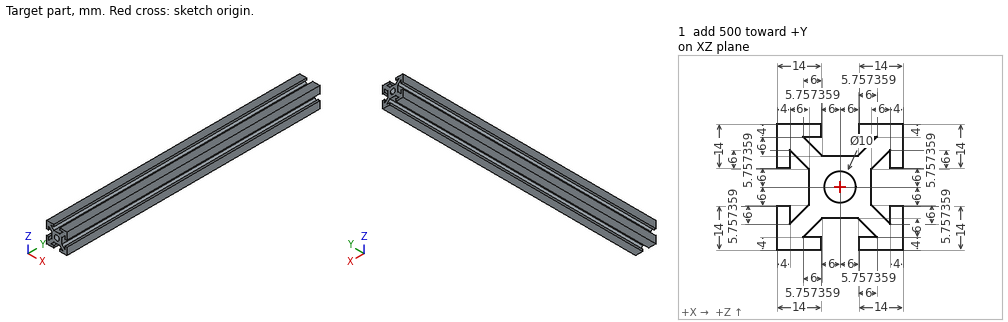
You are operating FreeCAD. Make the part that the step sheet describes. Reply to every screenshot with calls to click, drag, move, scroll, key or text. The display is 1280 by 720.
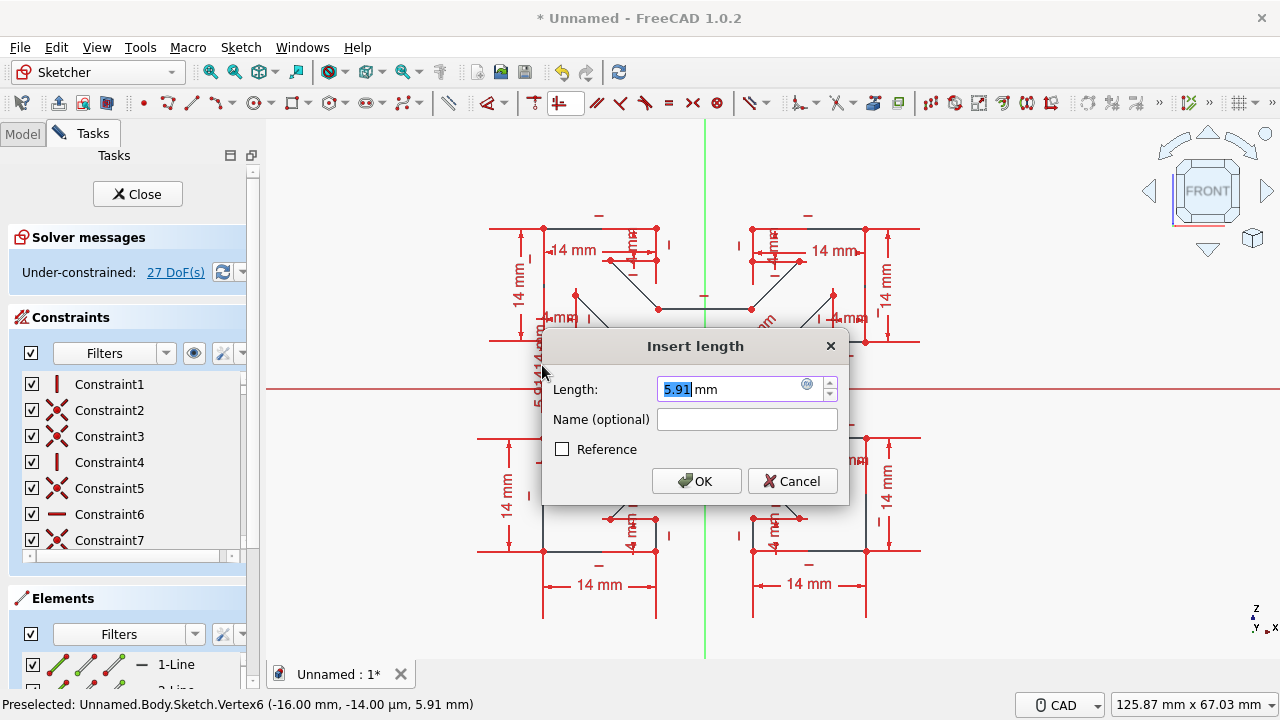
text(6)
key(Return)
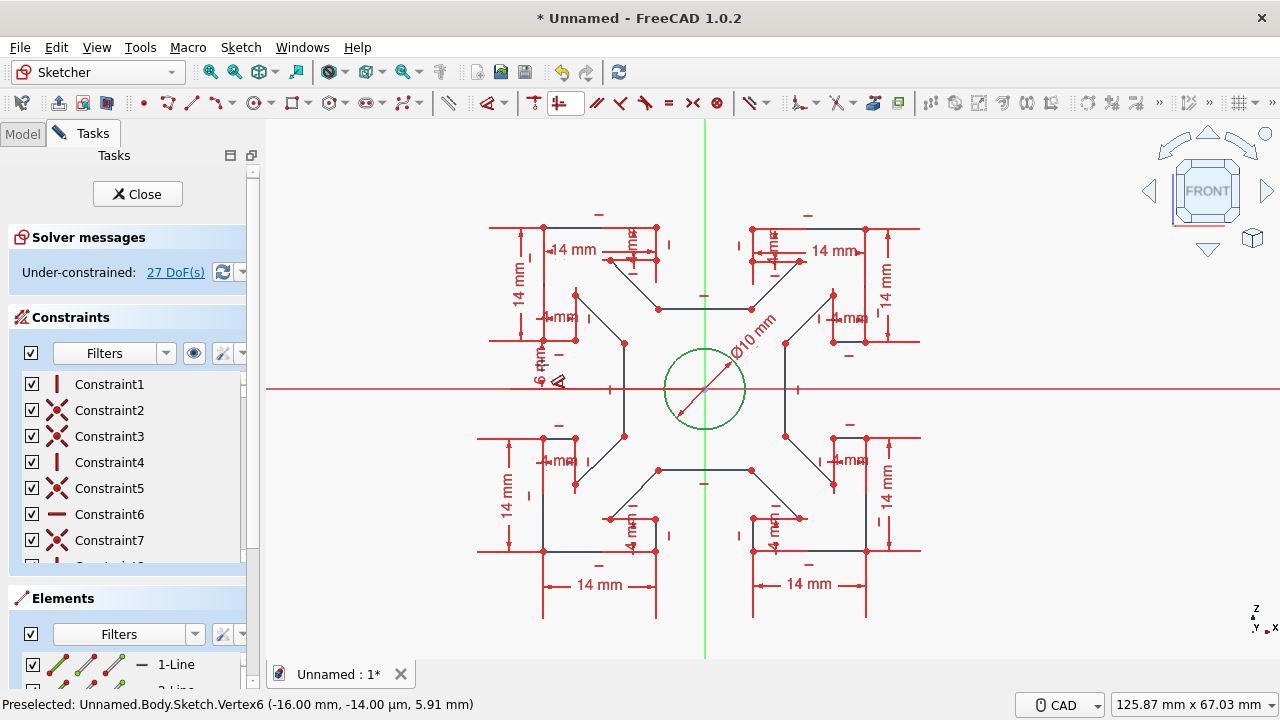
click(656, 228)
click(680, 194)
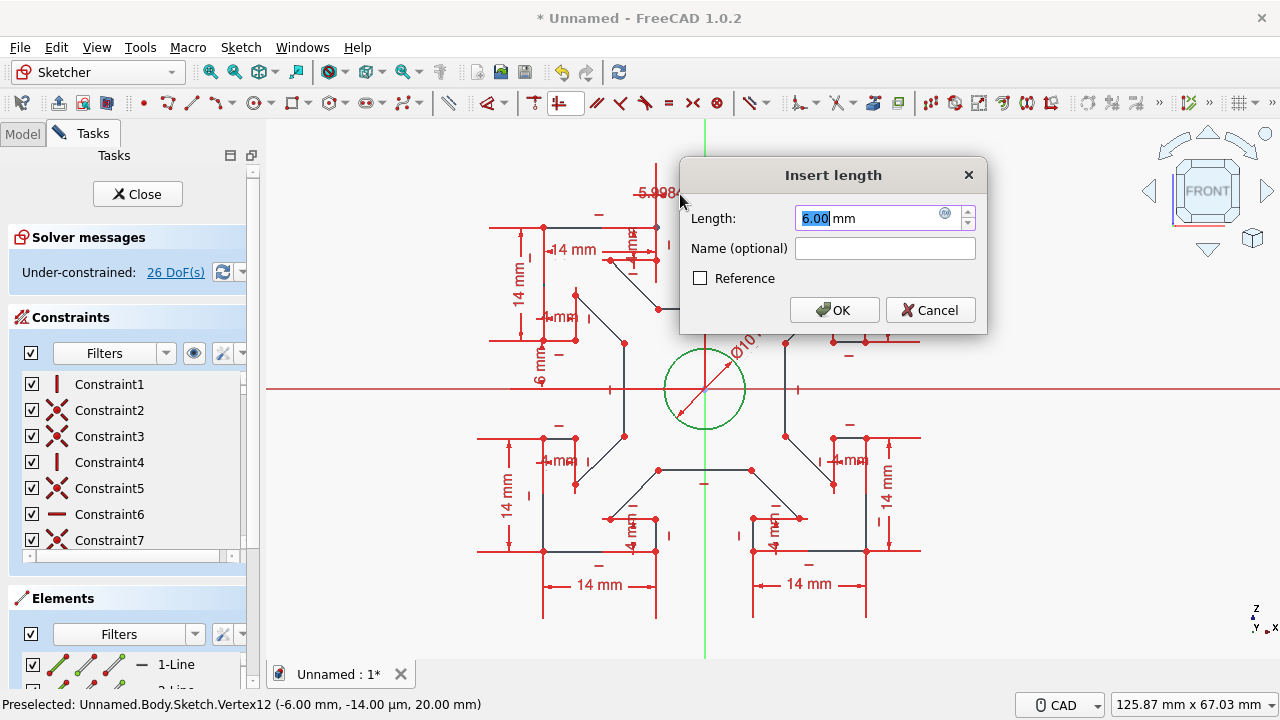
text(6)
key(Return)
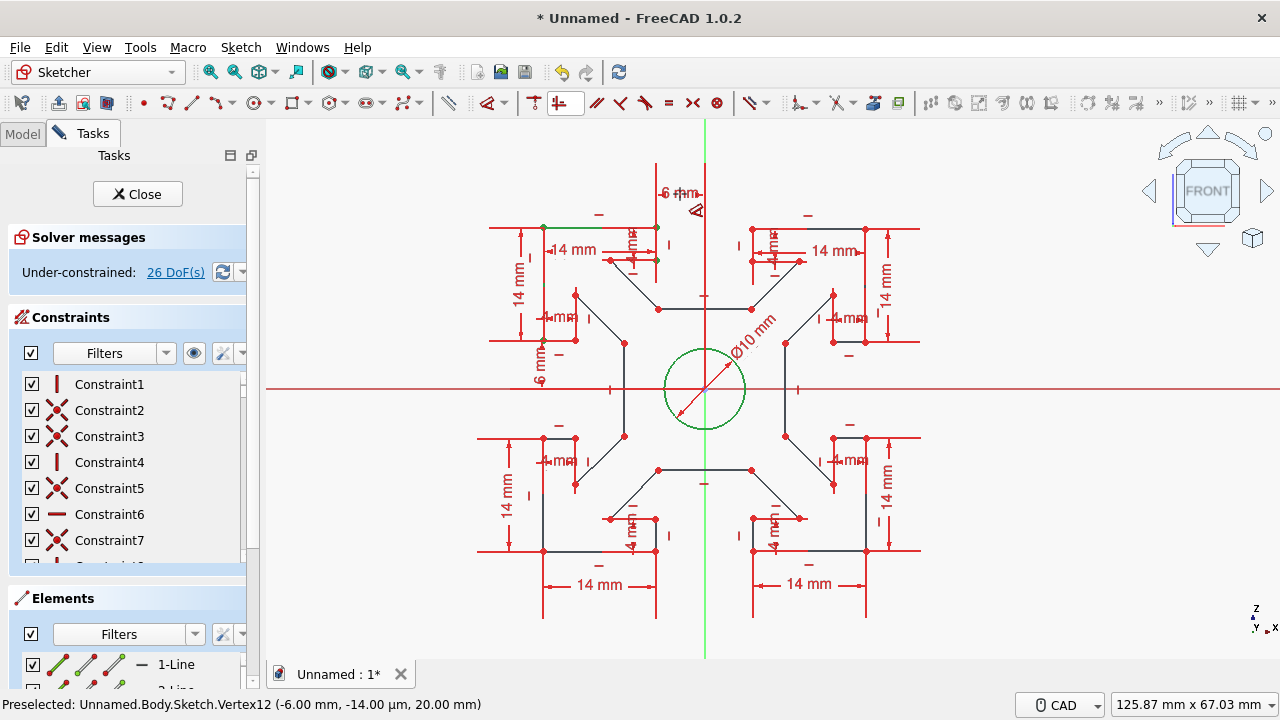
click(753, 262)
click(729, 447)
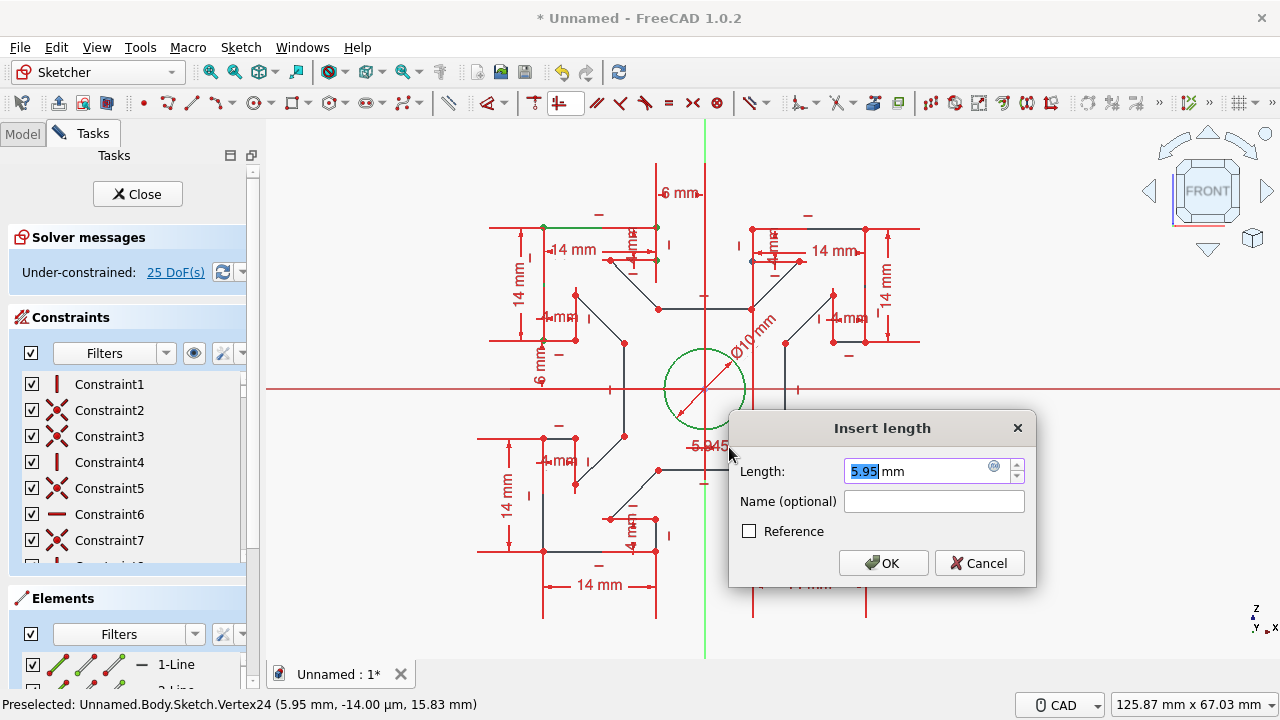
text(6)
key(Return)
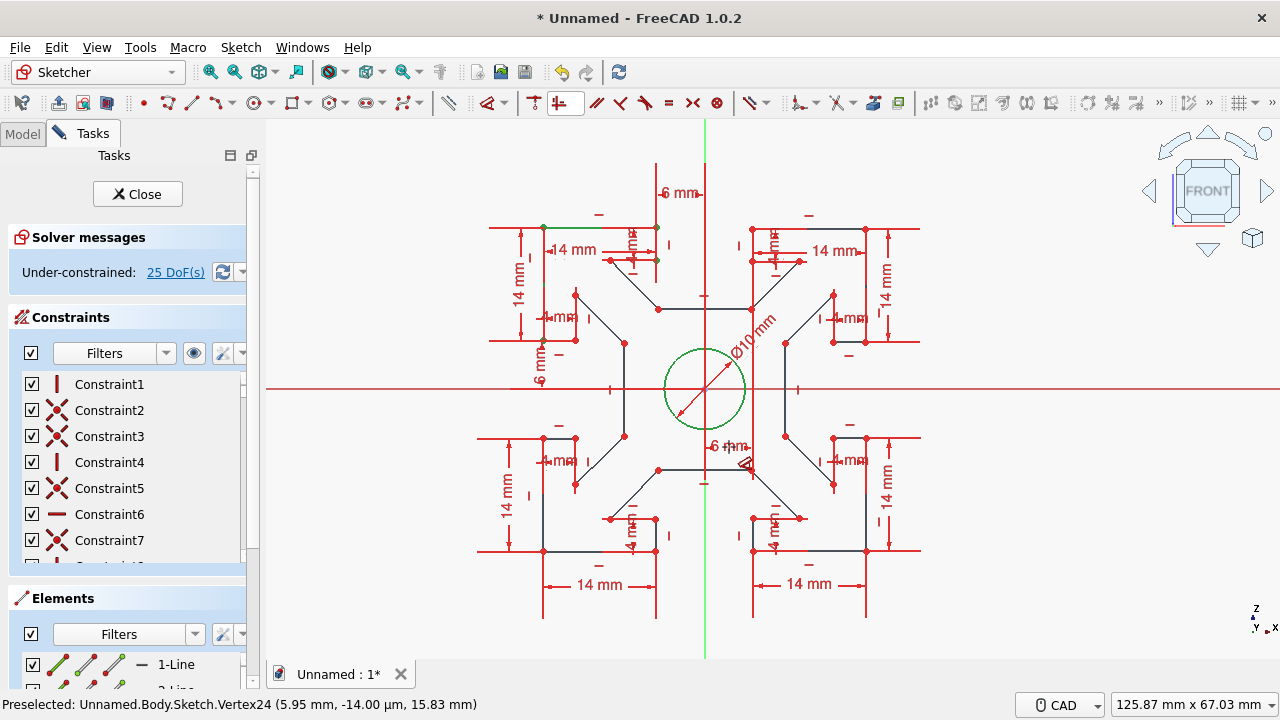
click(866, 342)
click(900, 366)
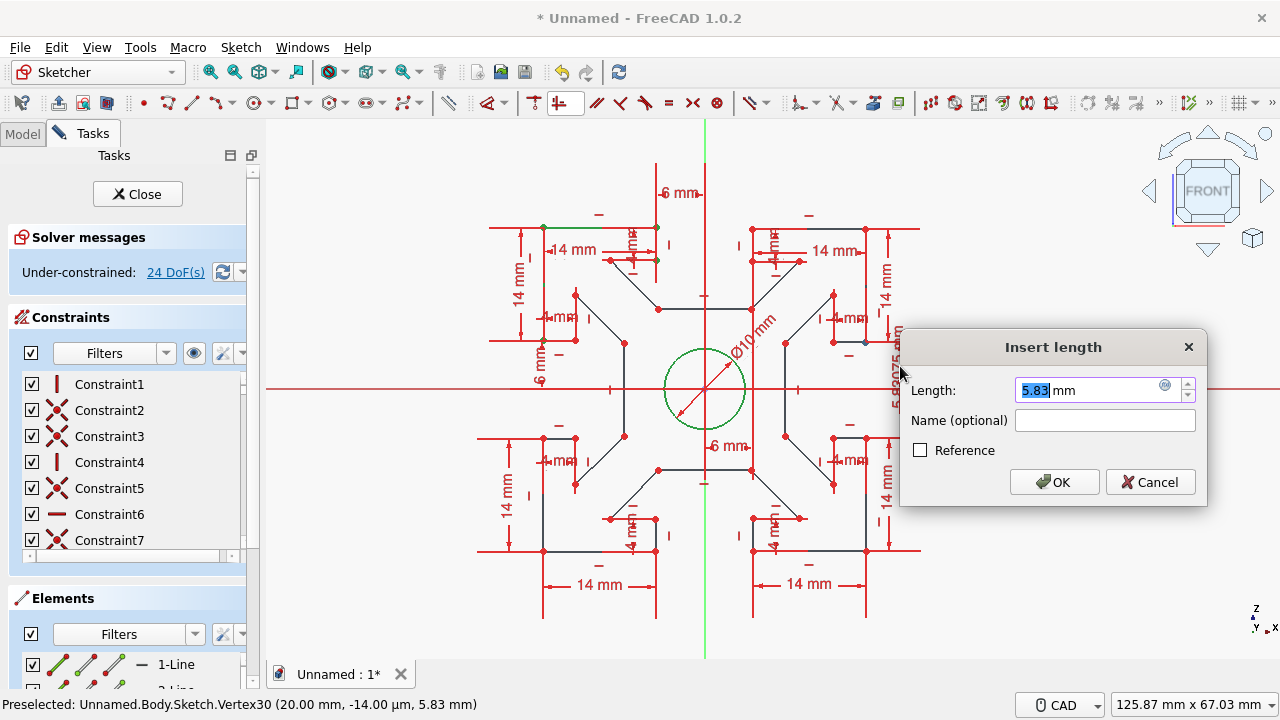
text(6)
key(Return)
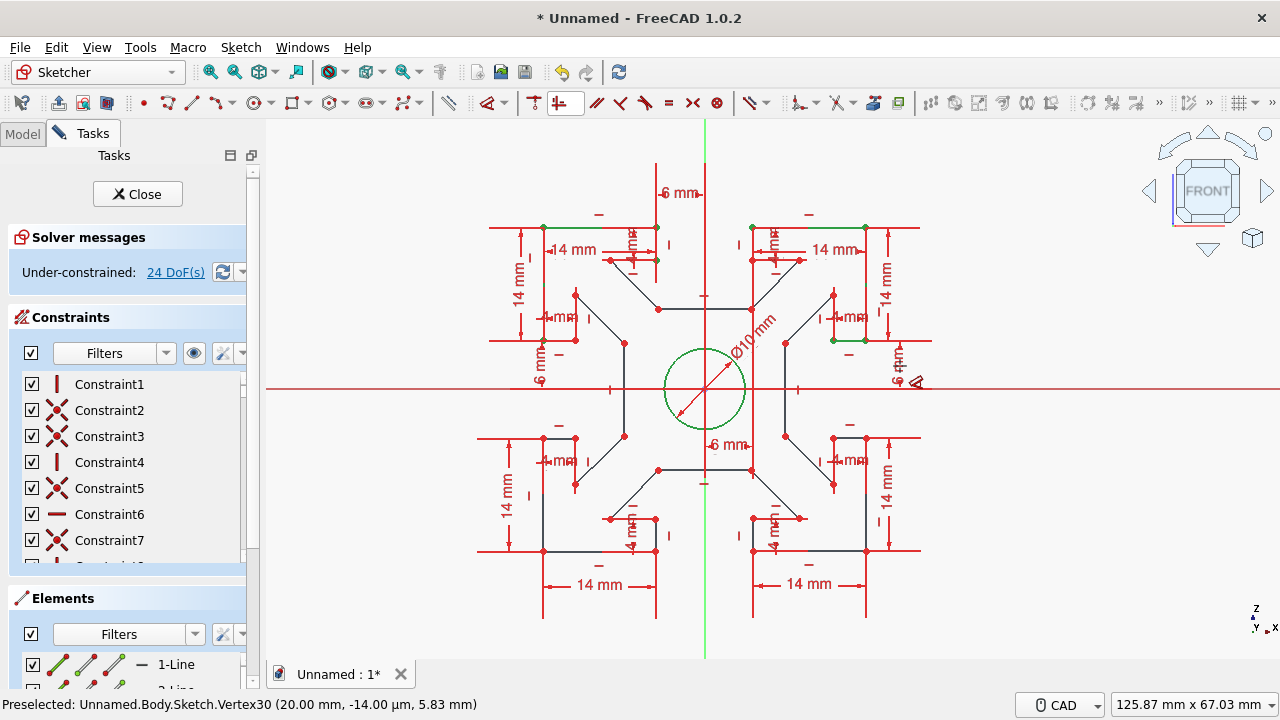
click(834, 438)
click(868, 414)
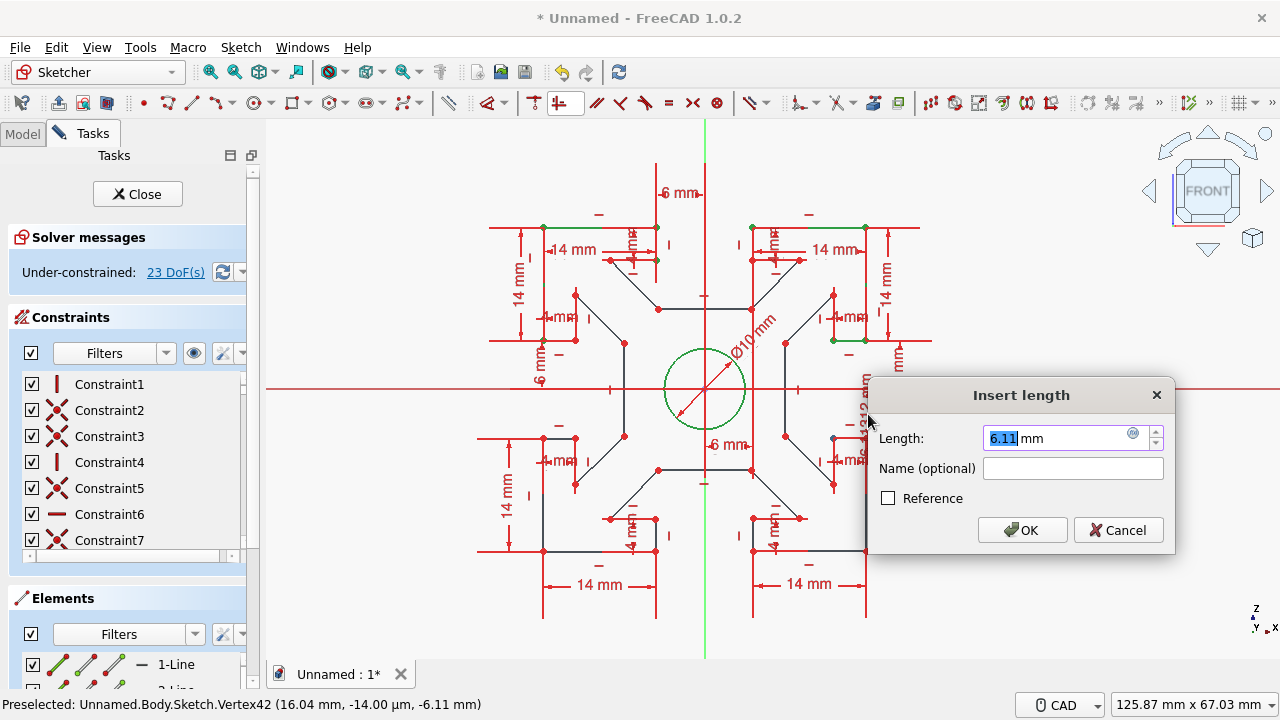
text(6)
key(Return)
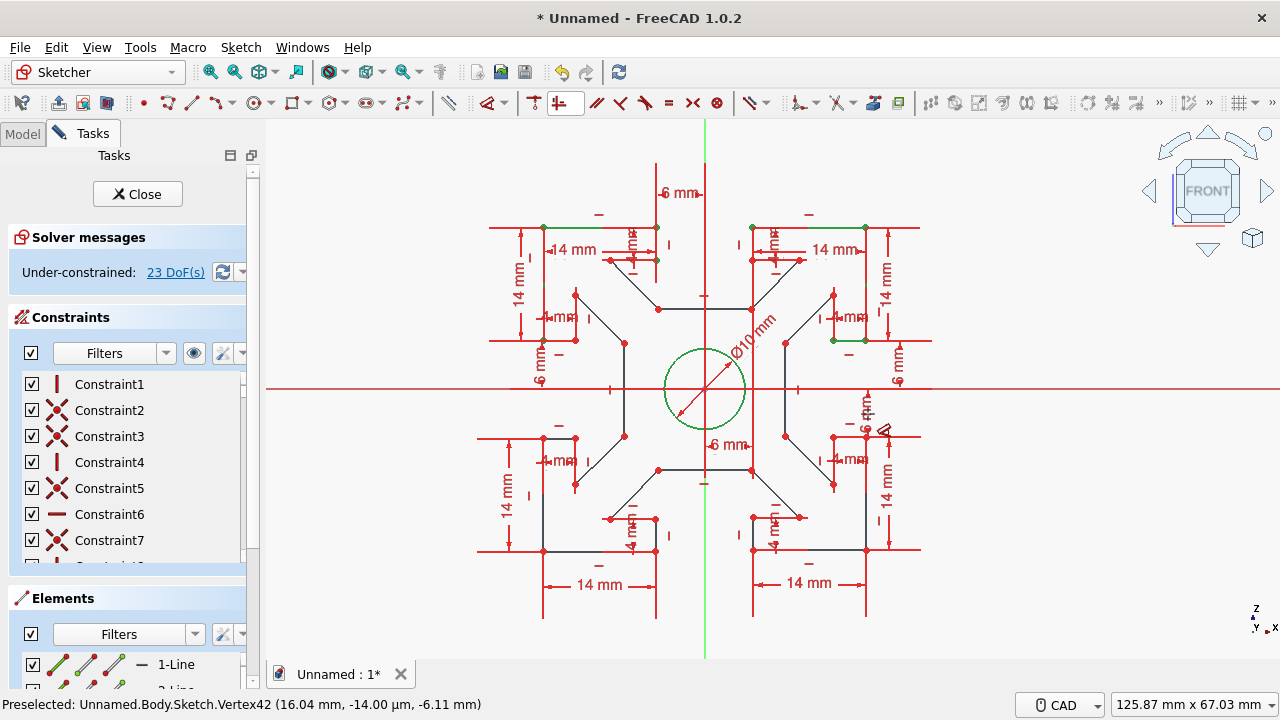
click(753, 550)
click(729, 584)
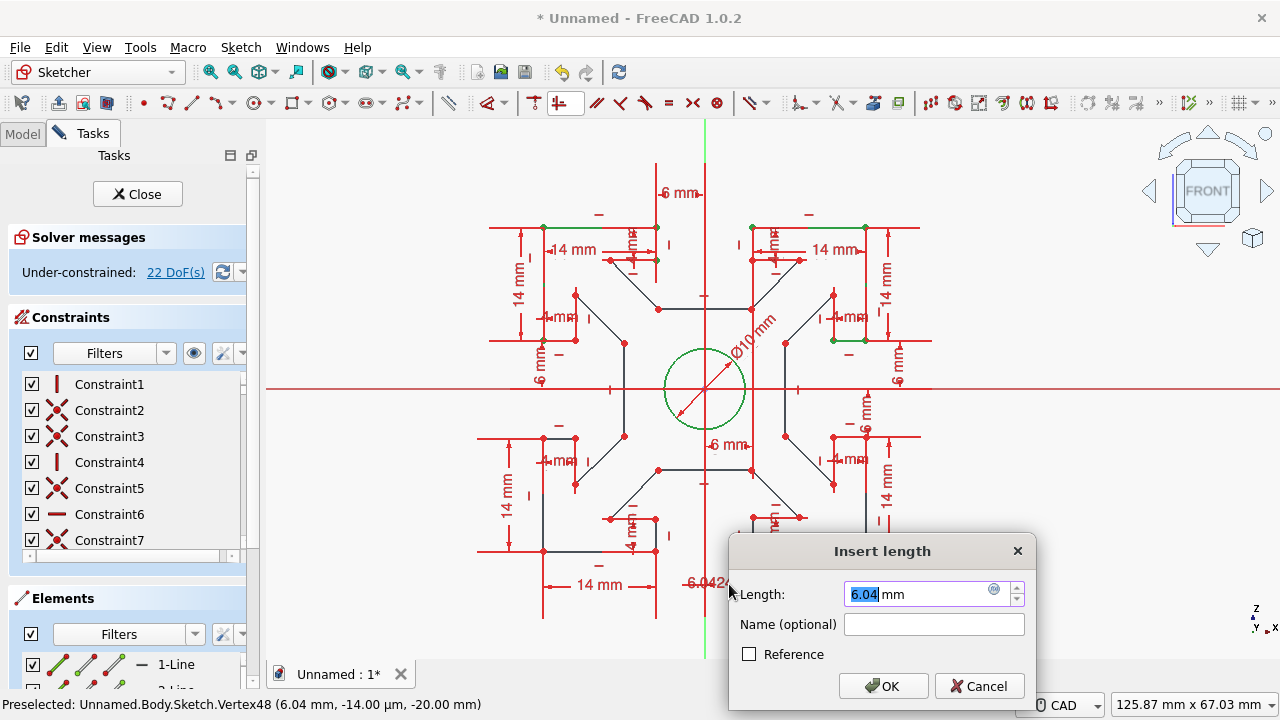
text(6)
key(Return)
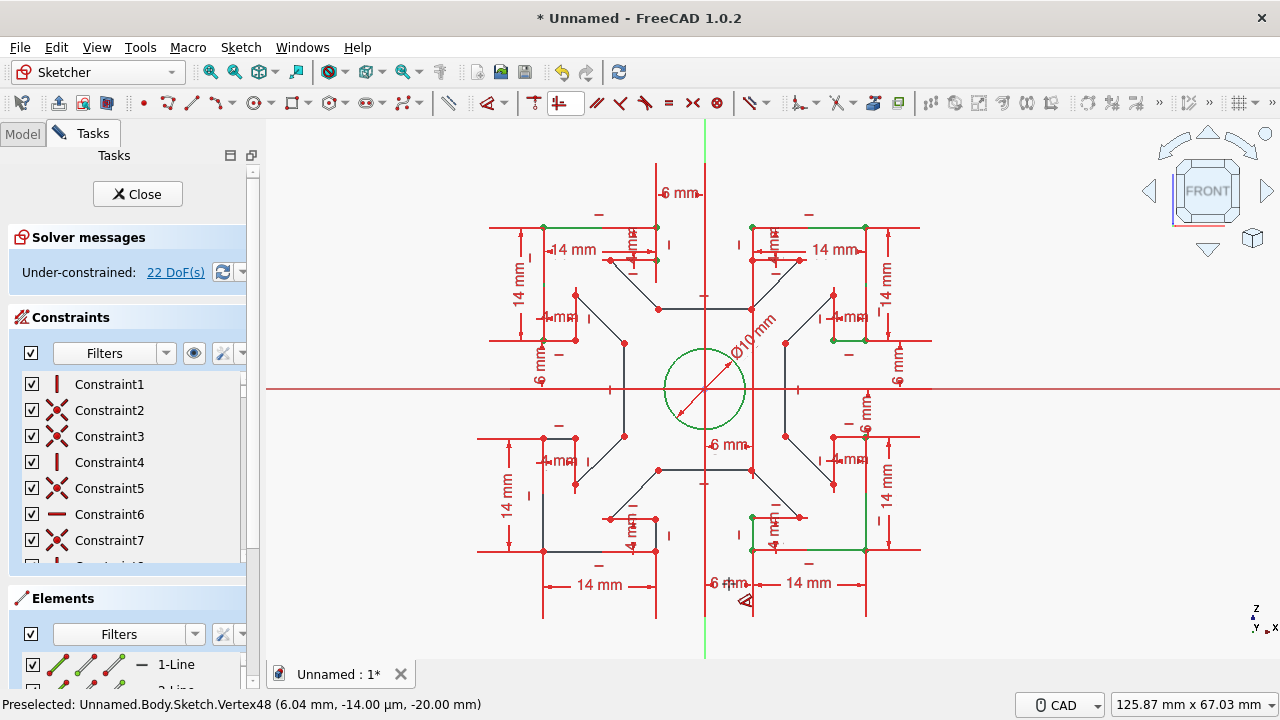
click(656, 519)
click(680, 553)